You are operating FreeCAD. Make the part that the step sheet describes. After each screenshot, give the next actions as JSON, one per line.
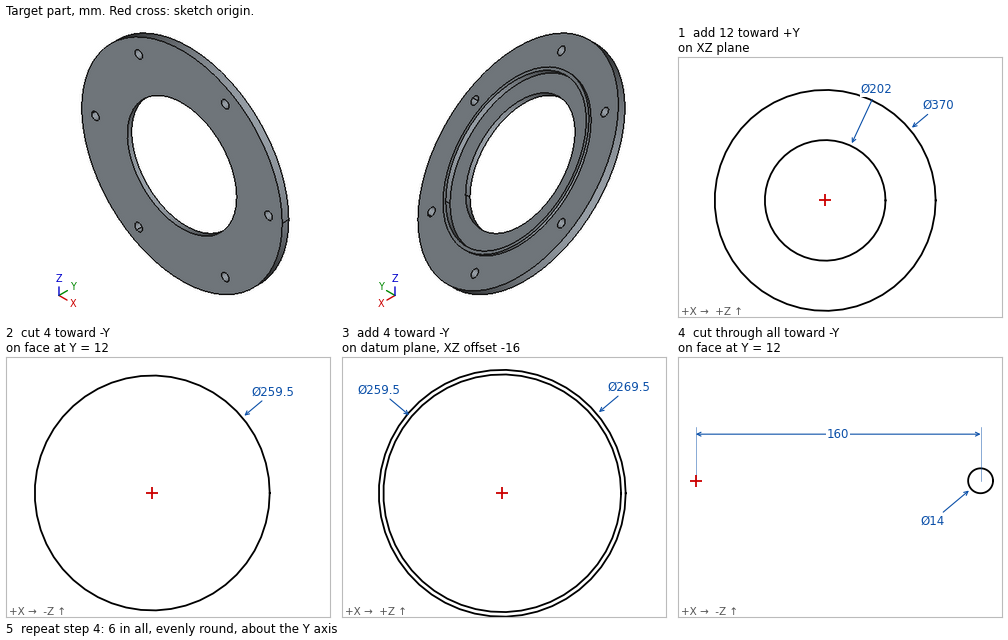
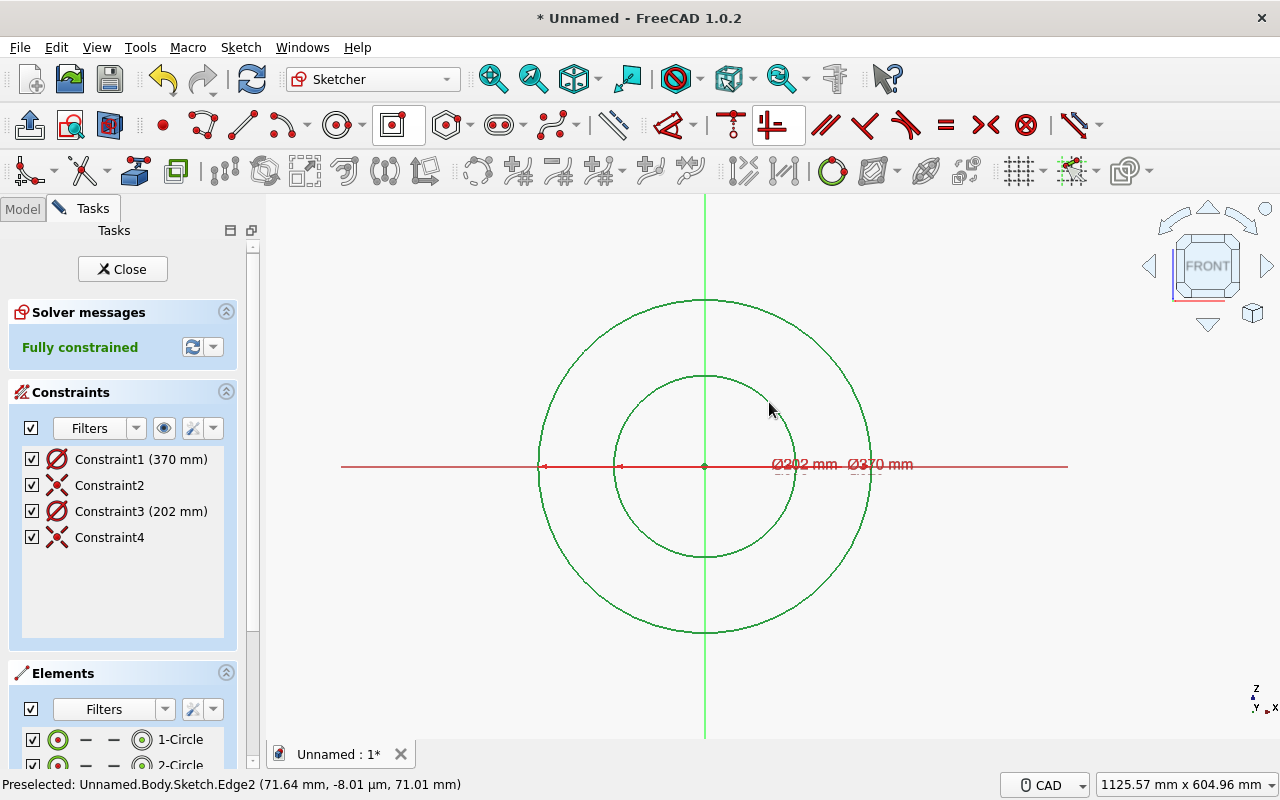
{"action": "left_click", "coordinate": [123, 269]}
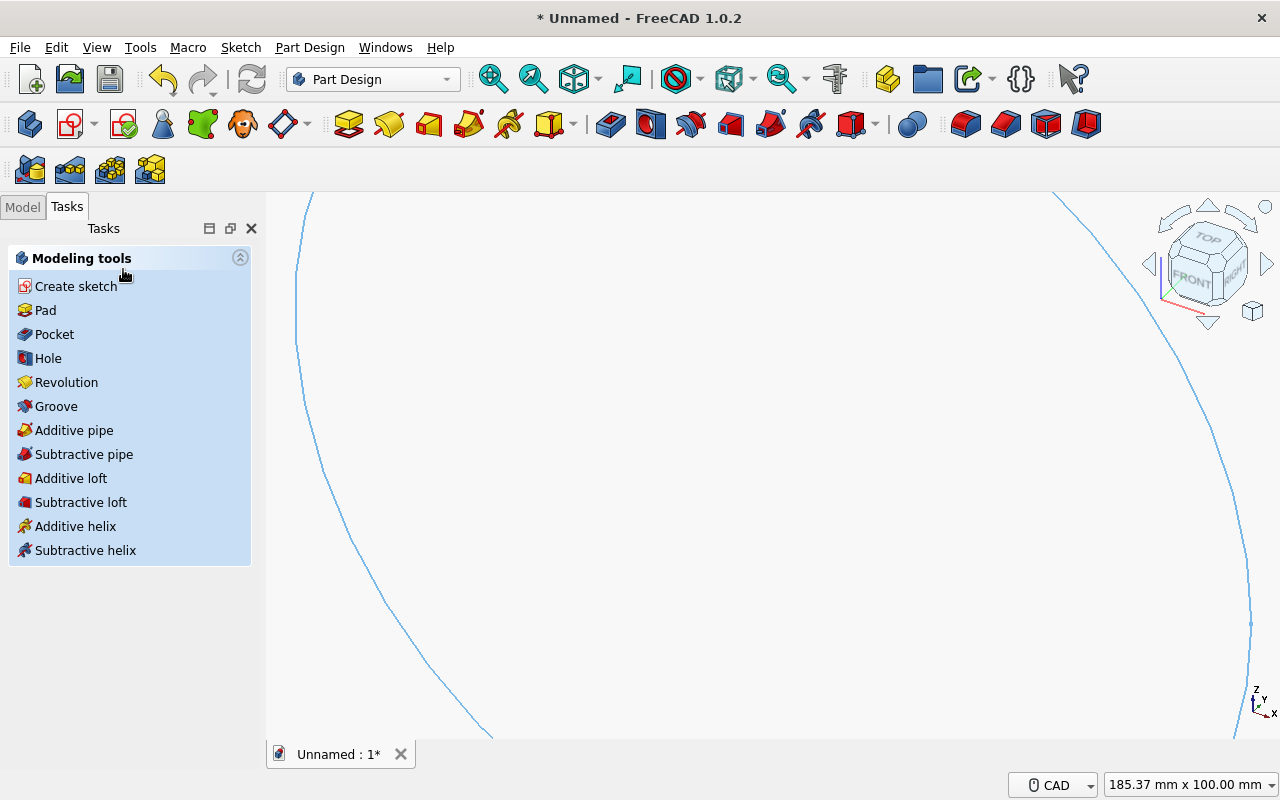
{"action": "left_click", "coordinate": [350, 124]}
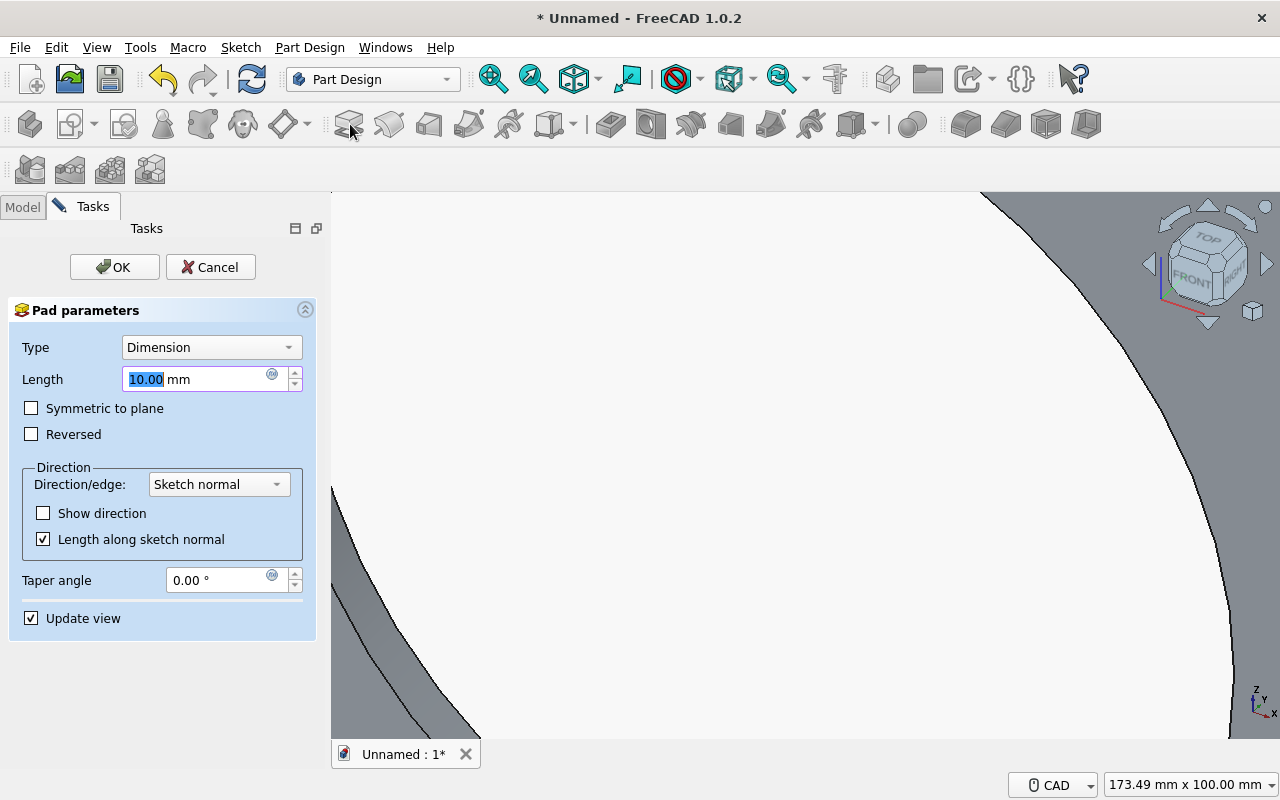
{"action": "type", "text": "12"}
{"action": "key", "text": "Tab"}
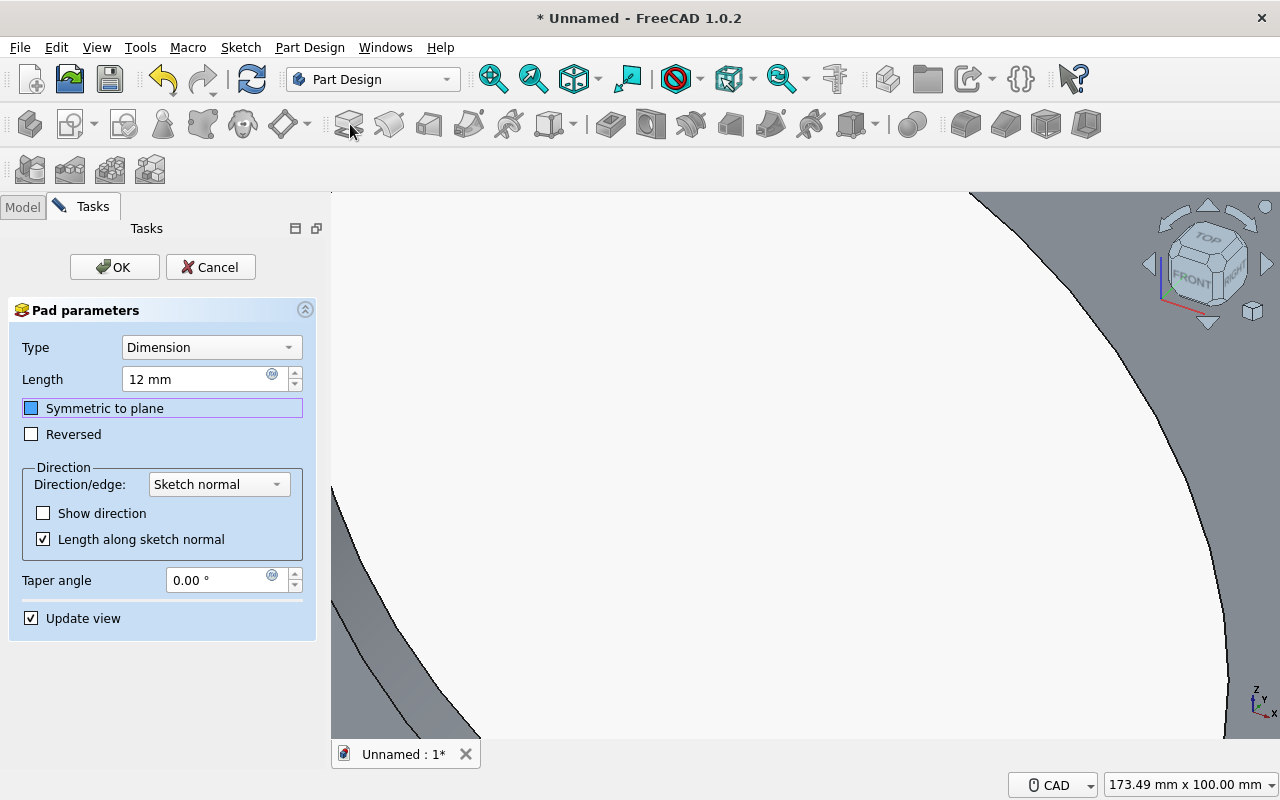
{"action": "left_click", "coordinate": [30, 434]}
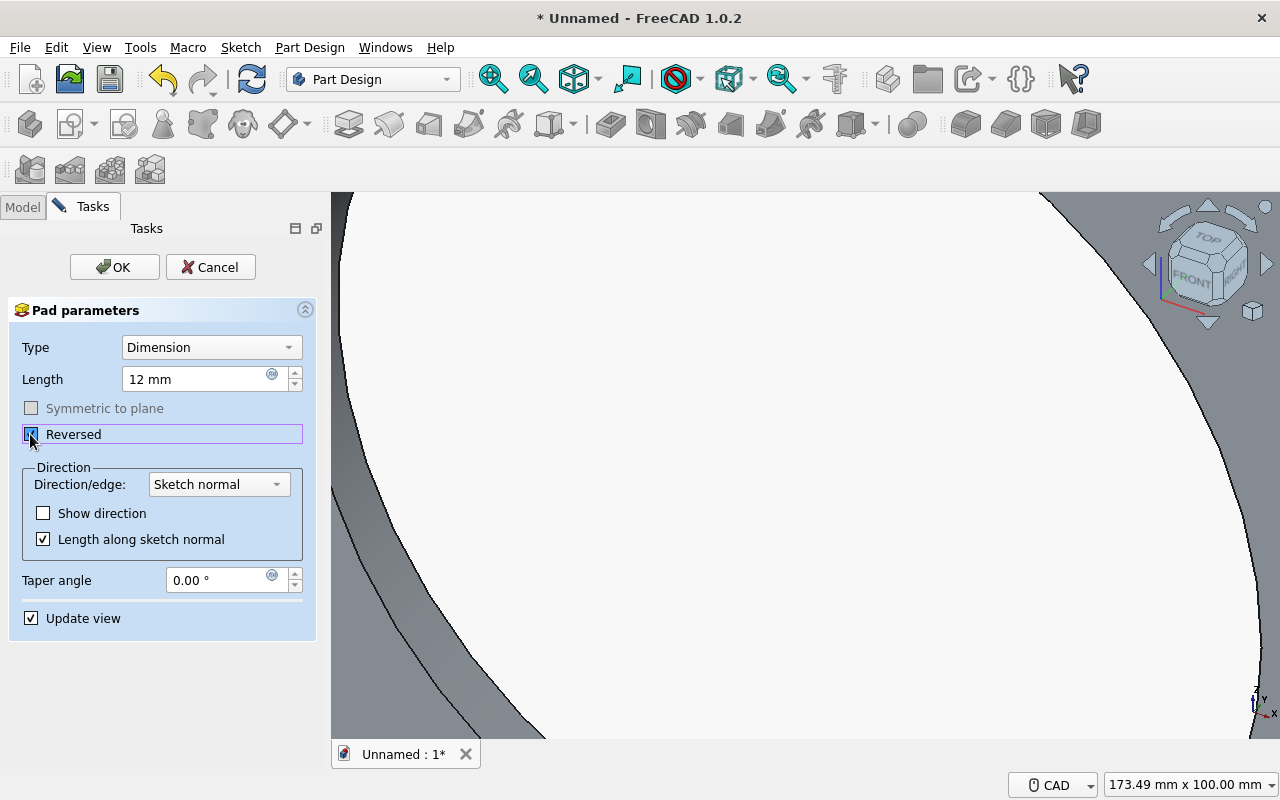
{"action": "left_click", "coordinate": [115, 267]}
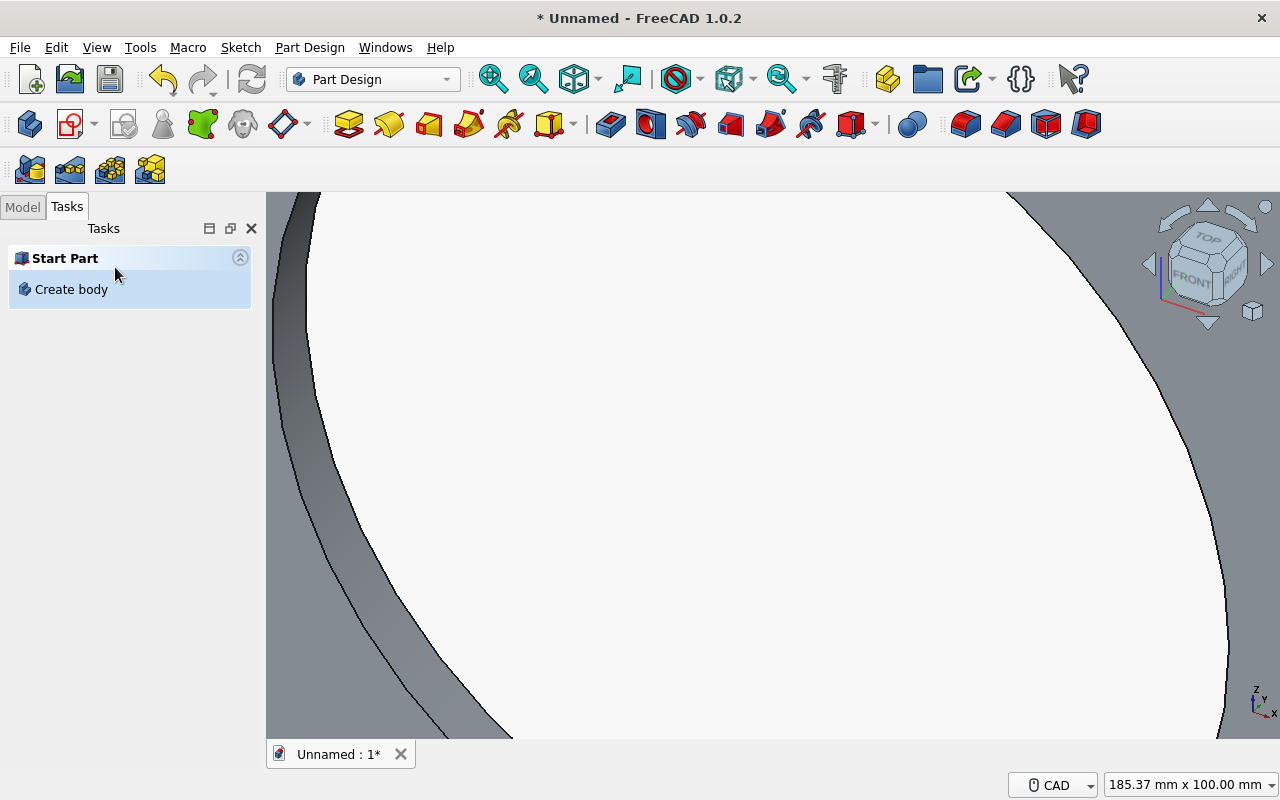
{"action": "left_click", "coordinate": [494, 80]}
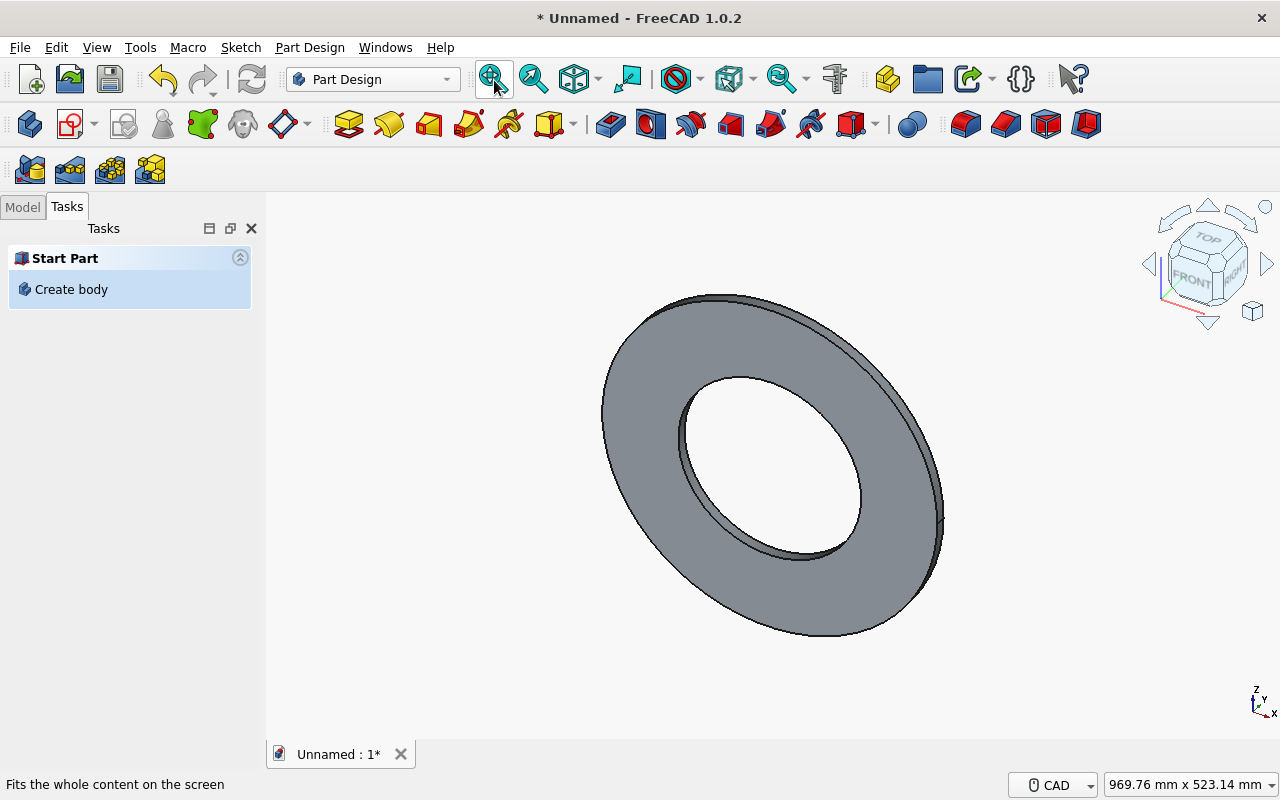
{"action": "key", "text": "4"}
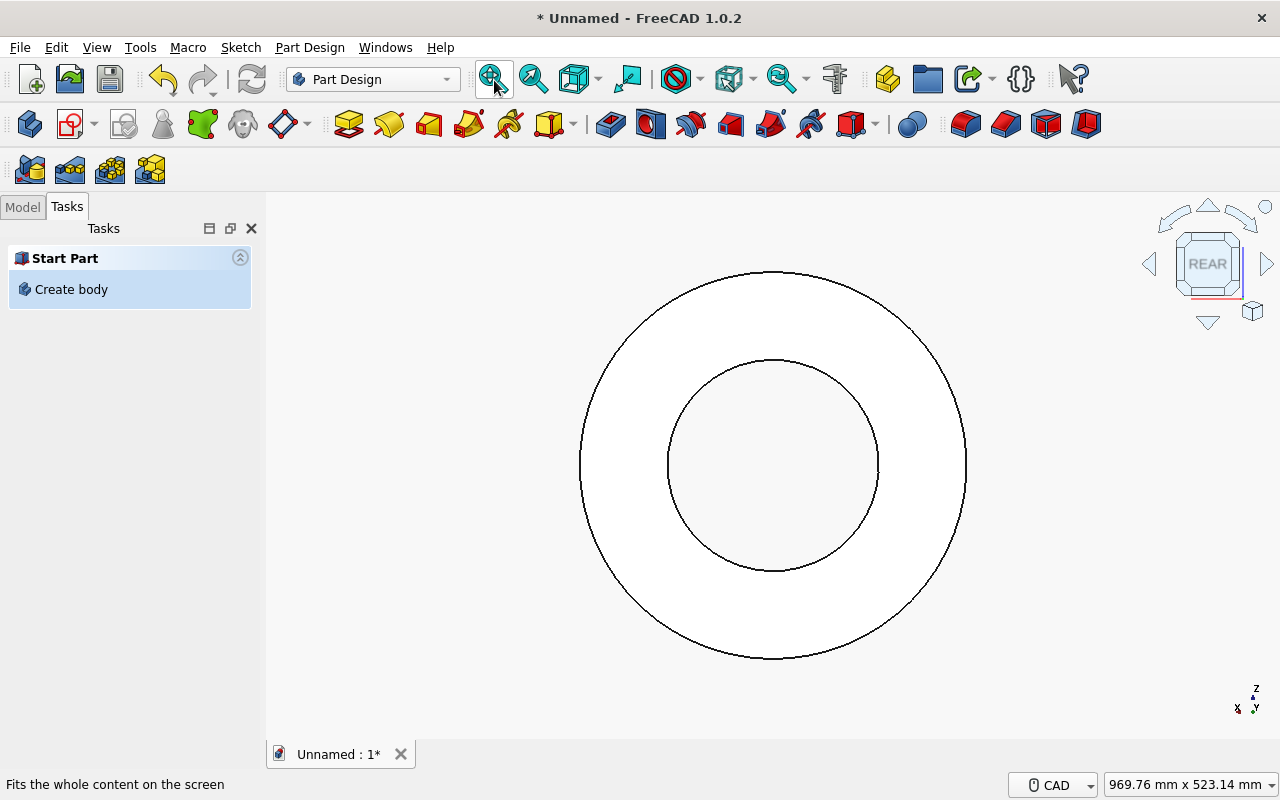
{"action": "left_click", "coordinate": [884, 575]}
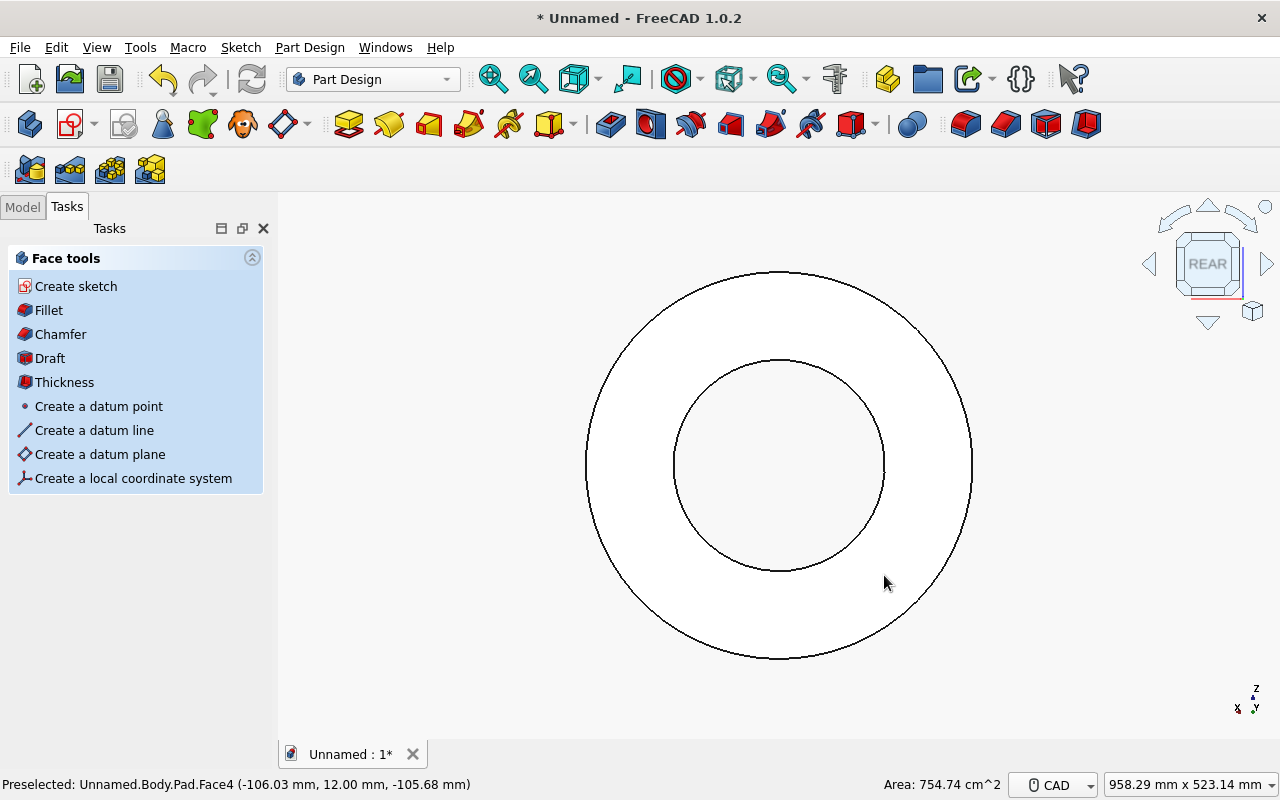
{"action": "left_click", "coordinate": [70, 124]}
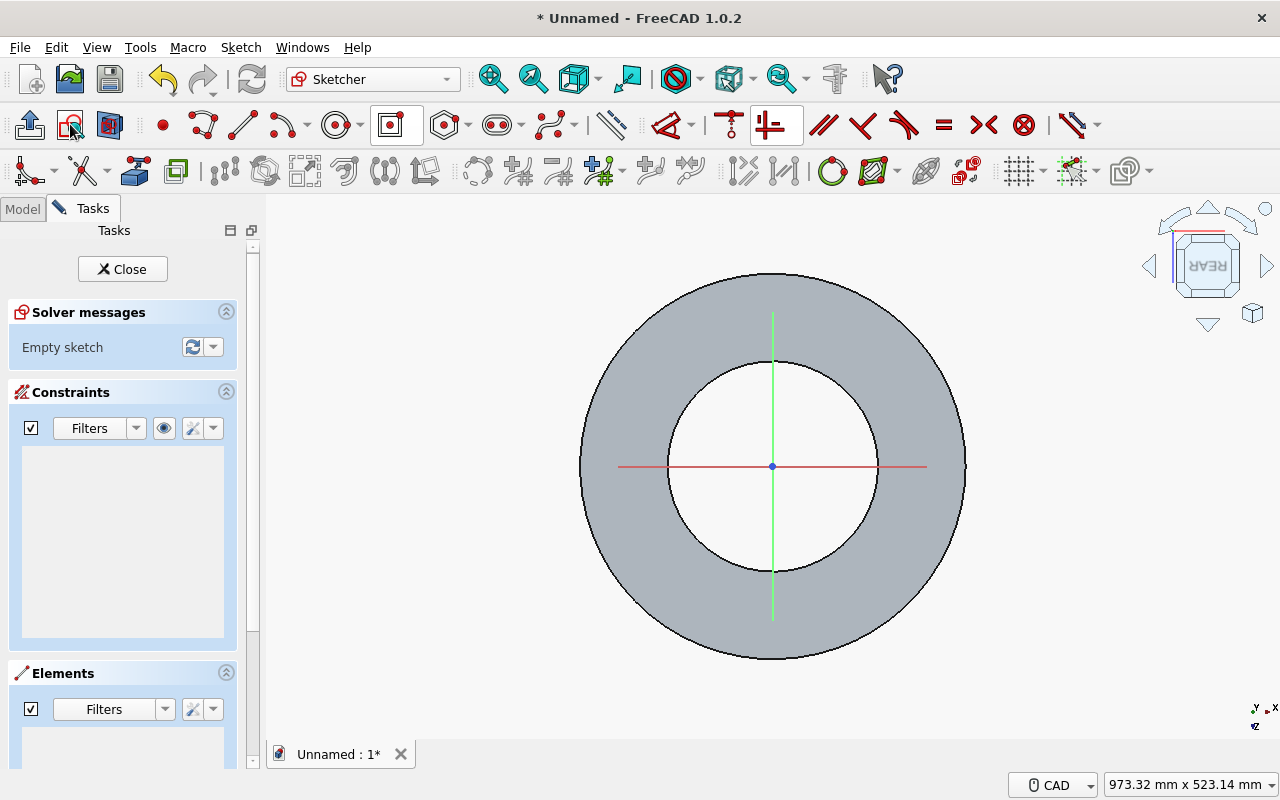
{"action": "left_click", "coordinate": [336, 126]}